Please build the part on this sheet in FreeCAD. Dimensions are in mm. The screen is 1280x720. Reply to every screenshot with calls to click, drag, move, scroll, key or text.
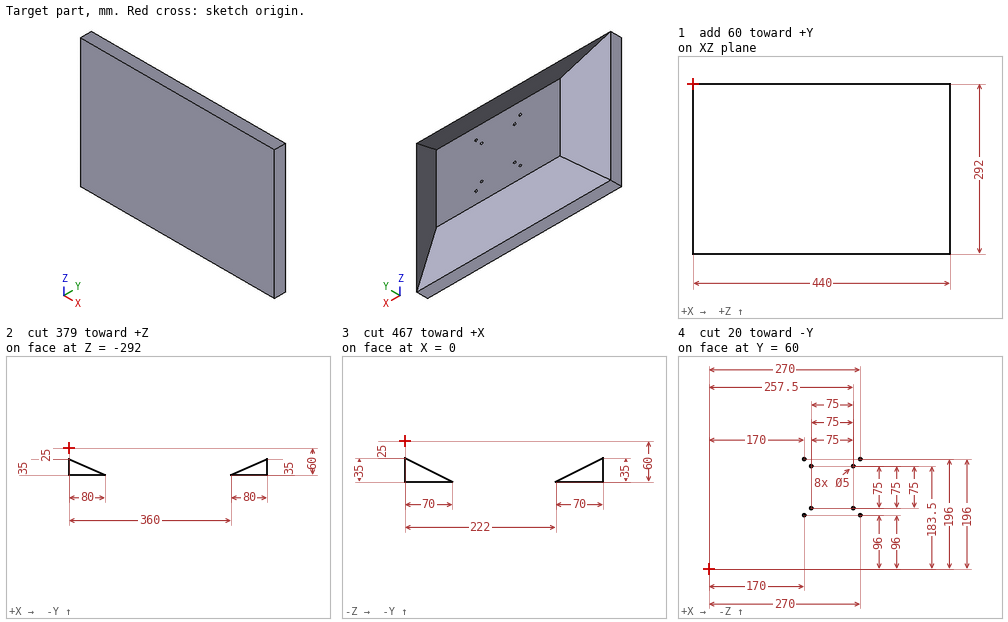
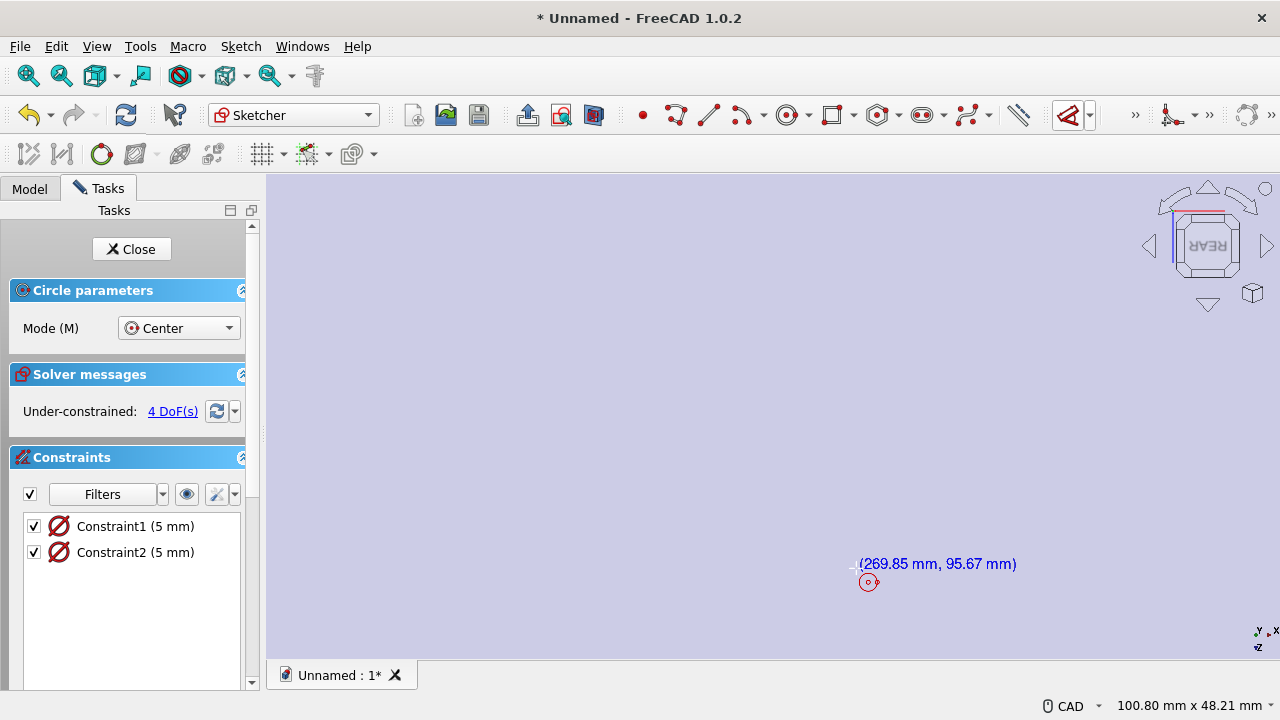
click(856, 566)
move(874, 548)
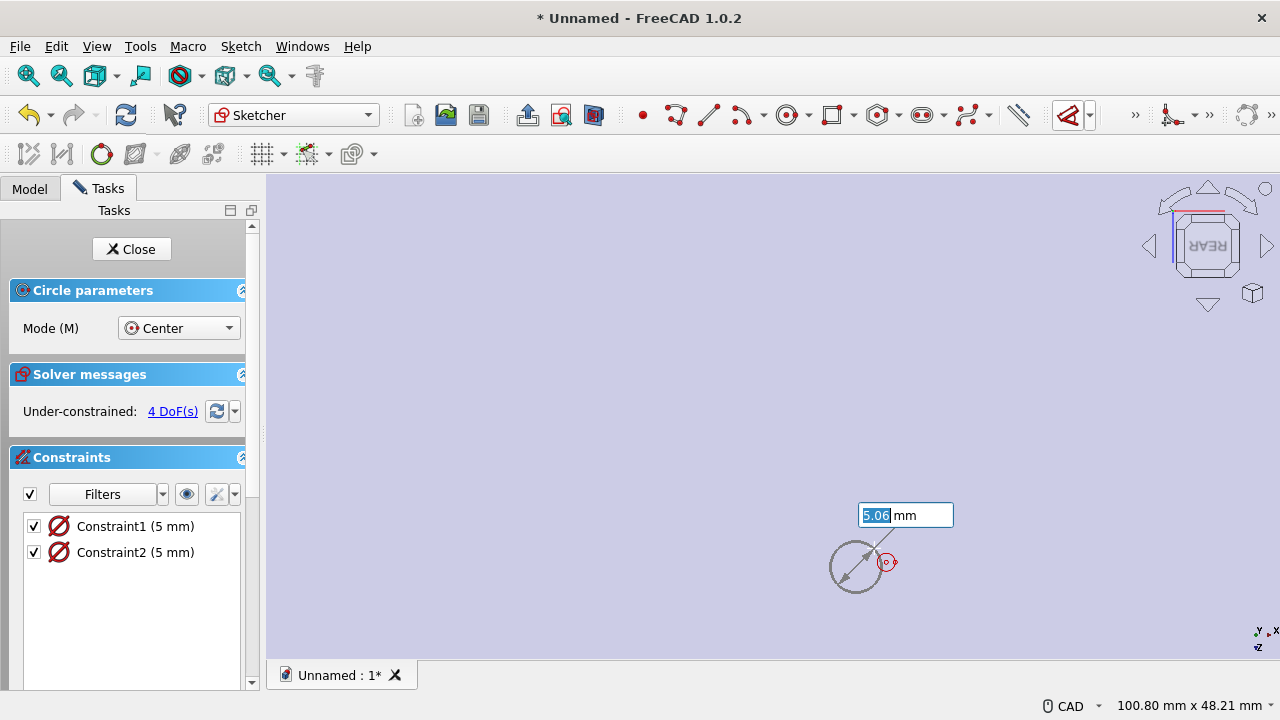
text(5)
key(Return)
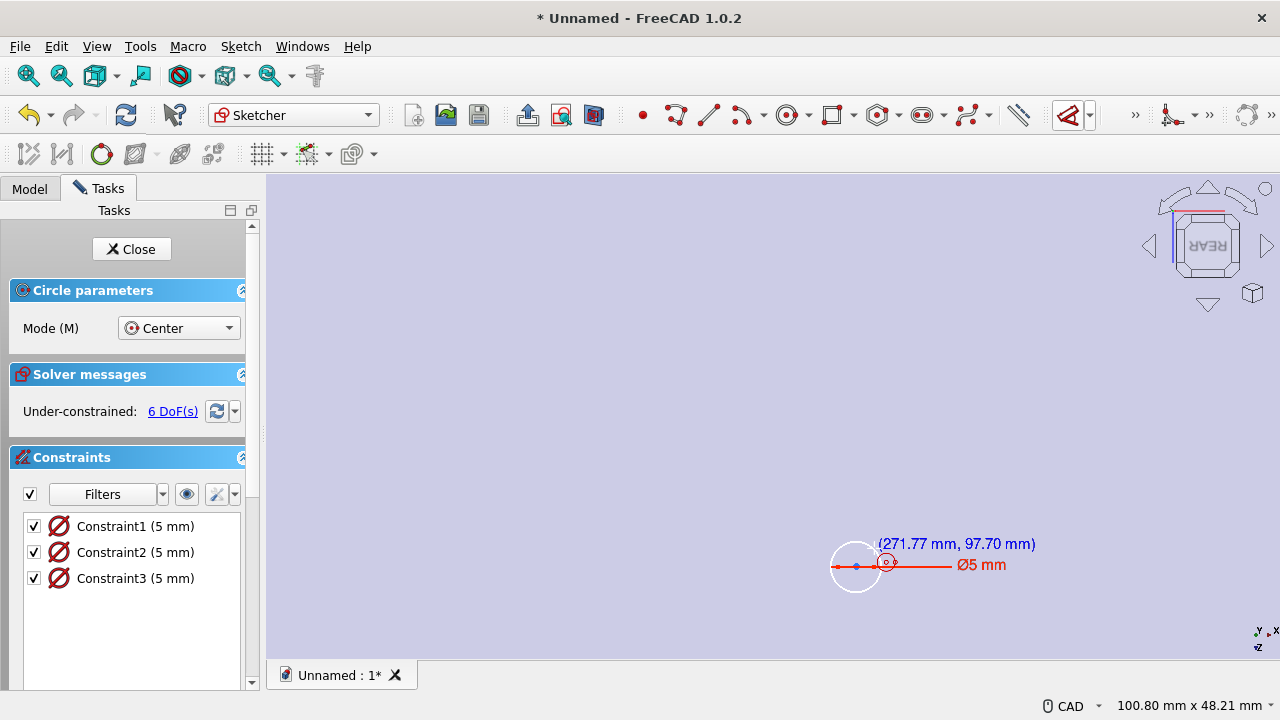
click(730, 440)
move(748, 423)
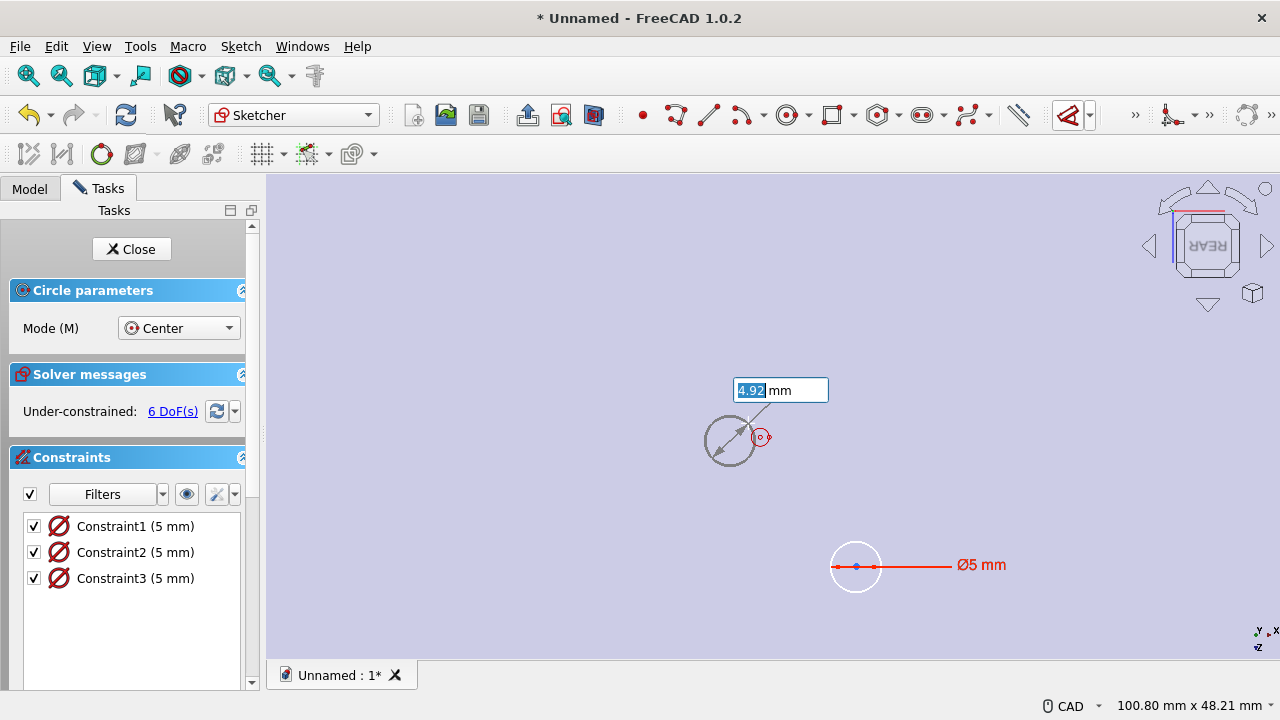
text(5)
key(Return)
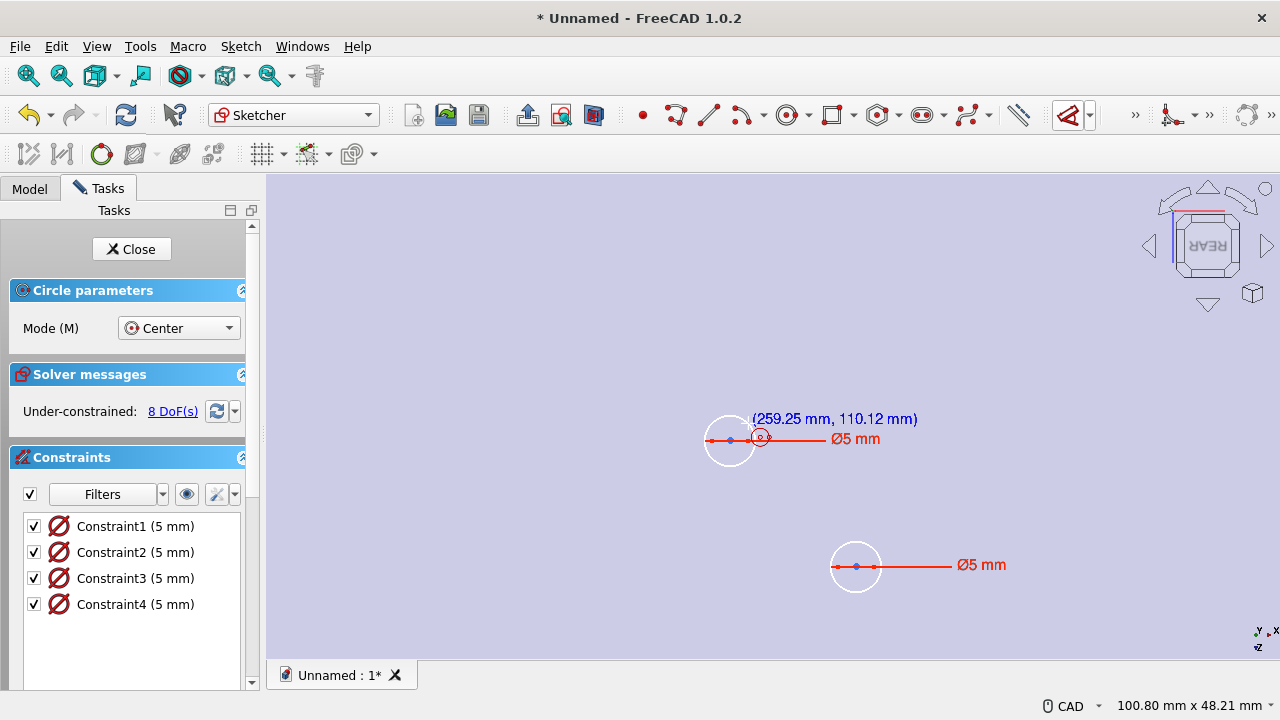
scroll(856, 569, down, 6)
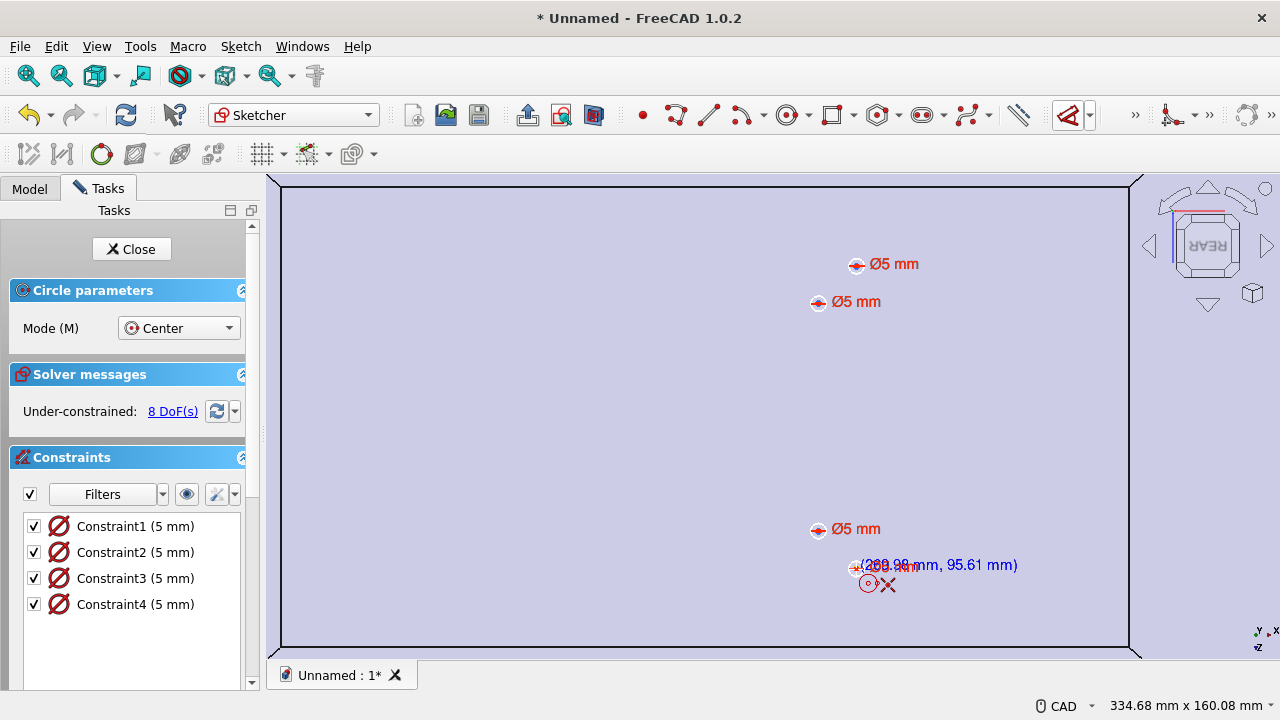
scroll(553, 569, up, 6)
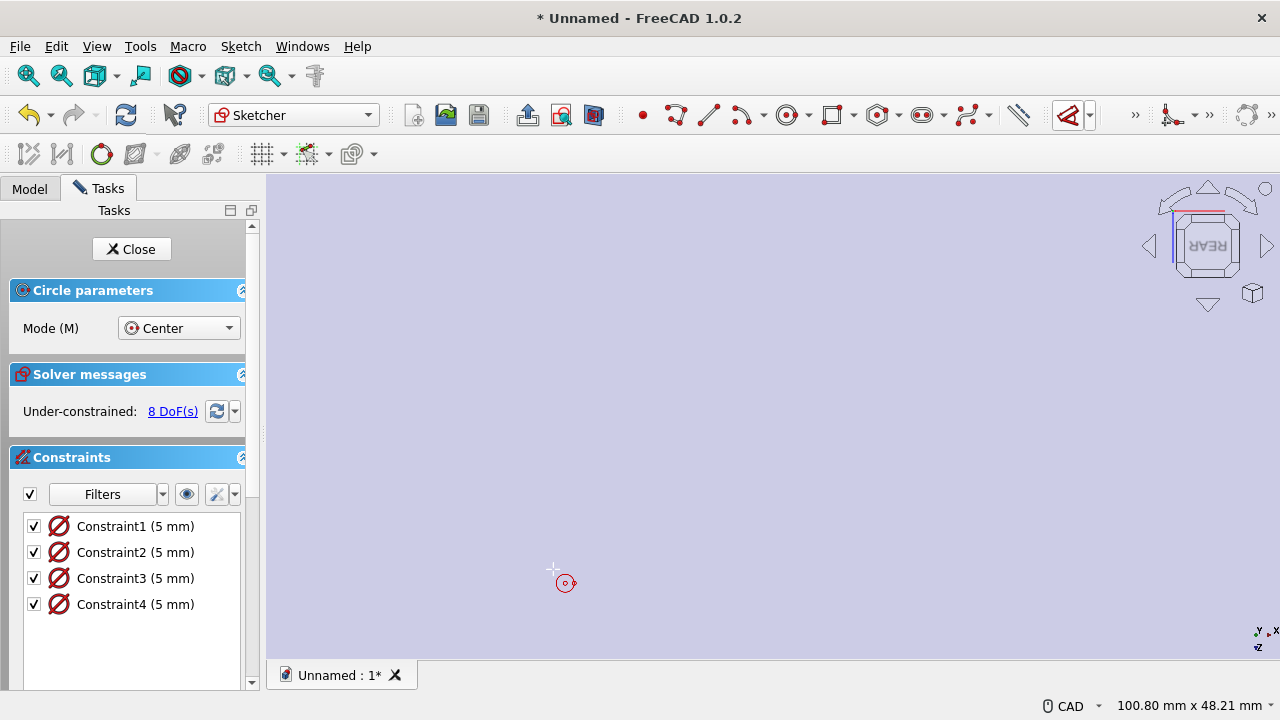
click(554, 566)
move(572, 548)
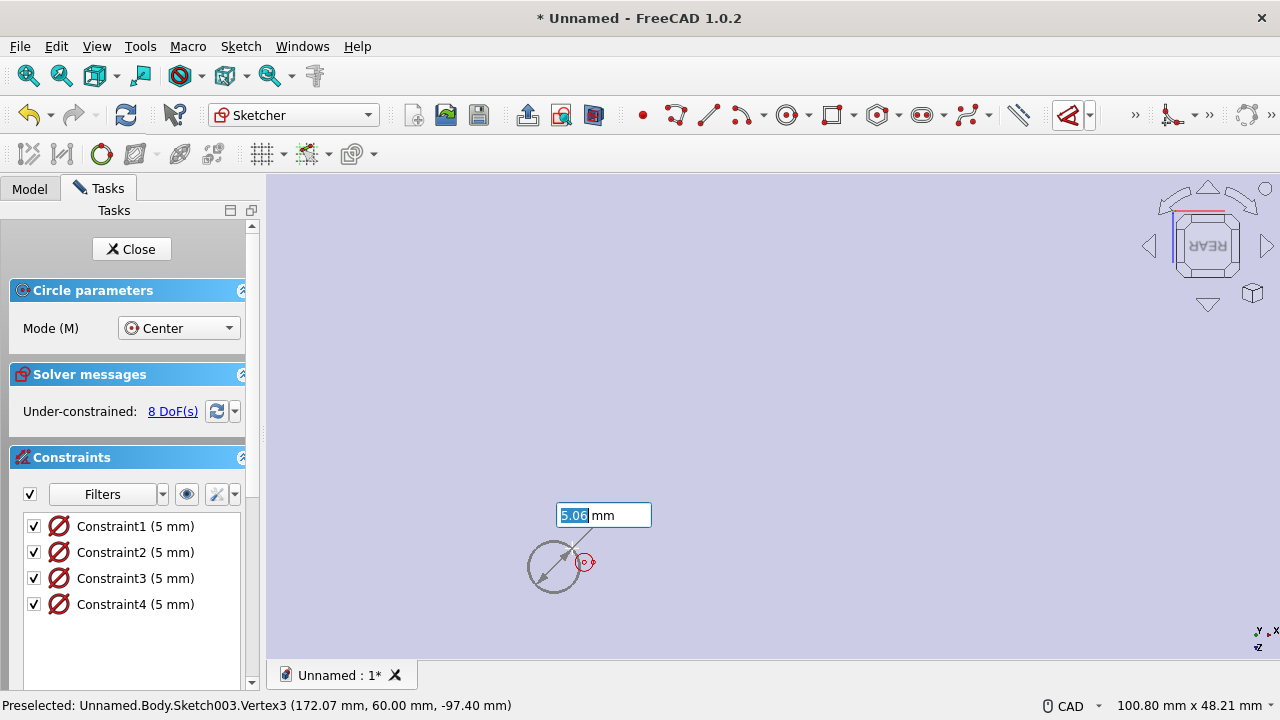
text(5)
key(Return)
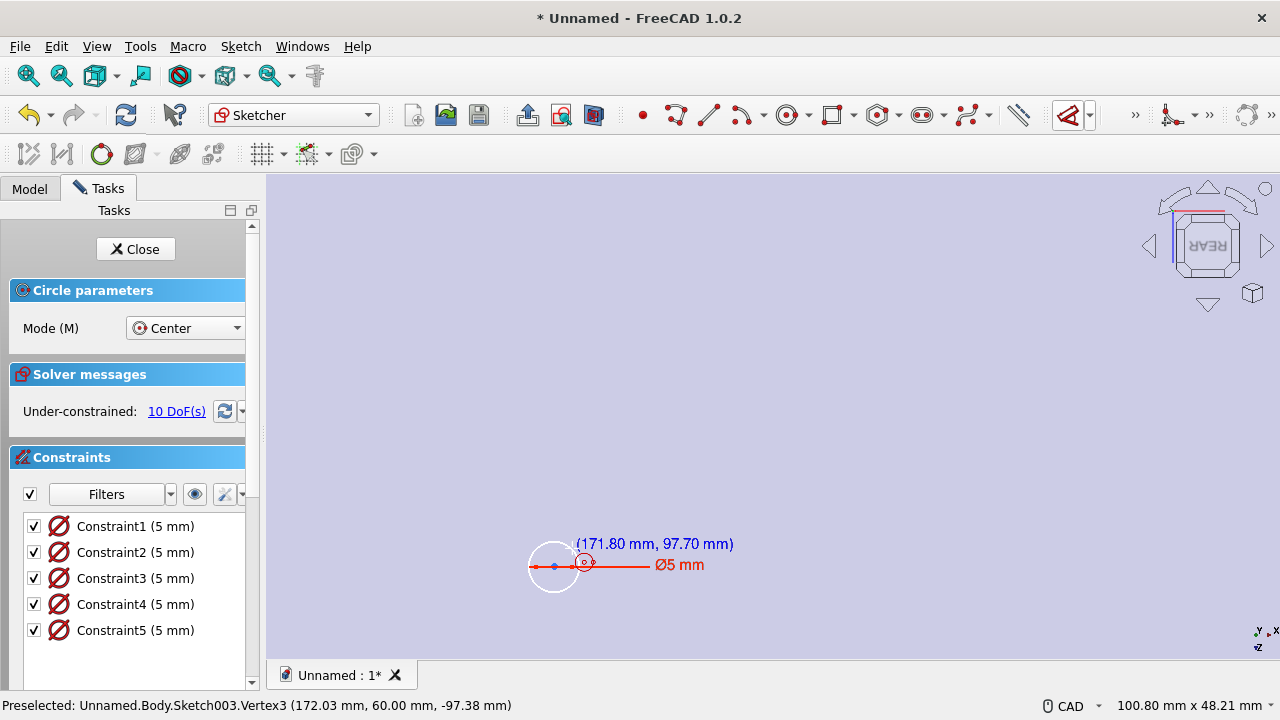
click(680, 440)
move(697, 423)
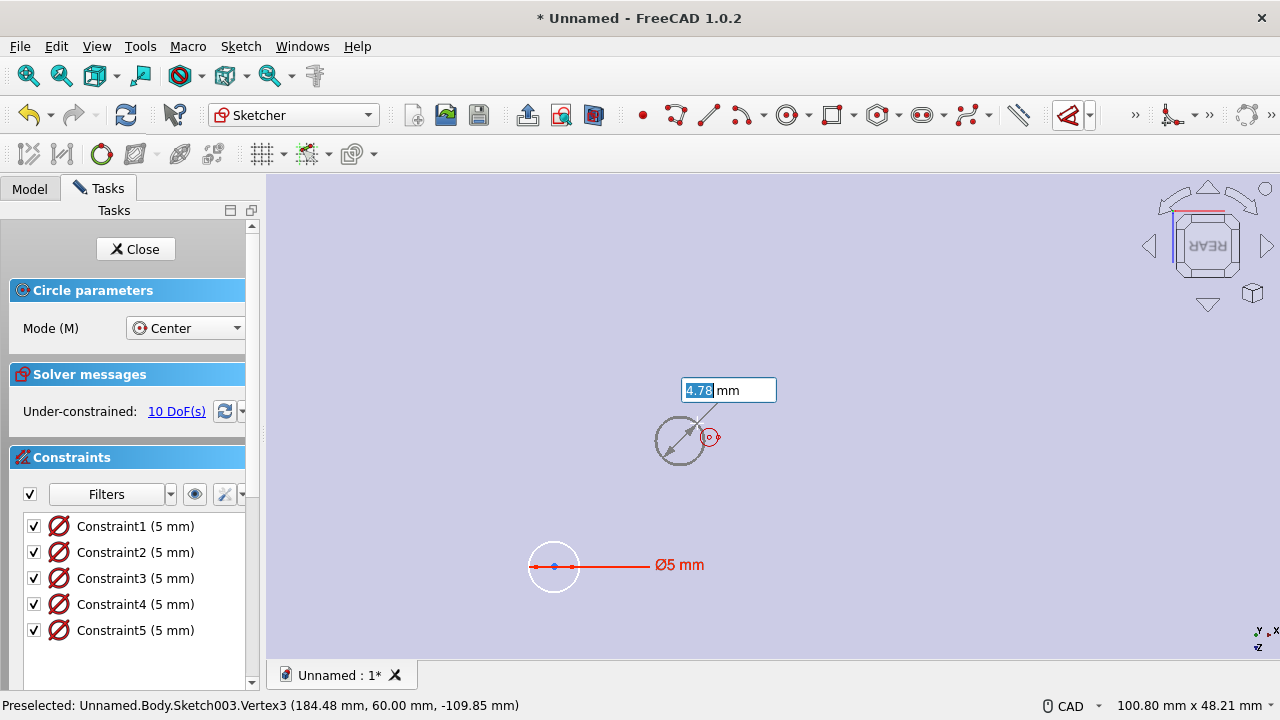
text(5)
key(Return)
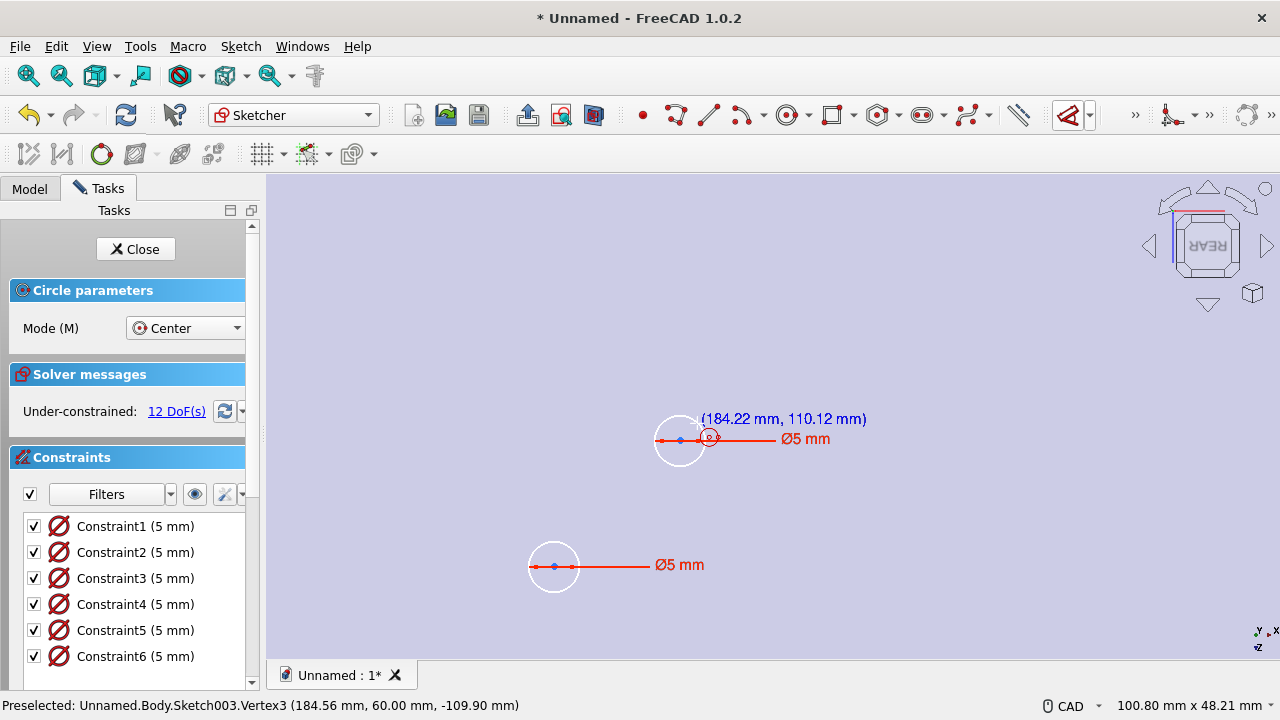
scroll(553, 569, down, 6)